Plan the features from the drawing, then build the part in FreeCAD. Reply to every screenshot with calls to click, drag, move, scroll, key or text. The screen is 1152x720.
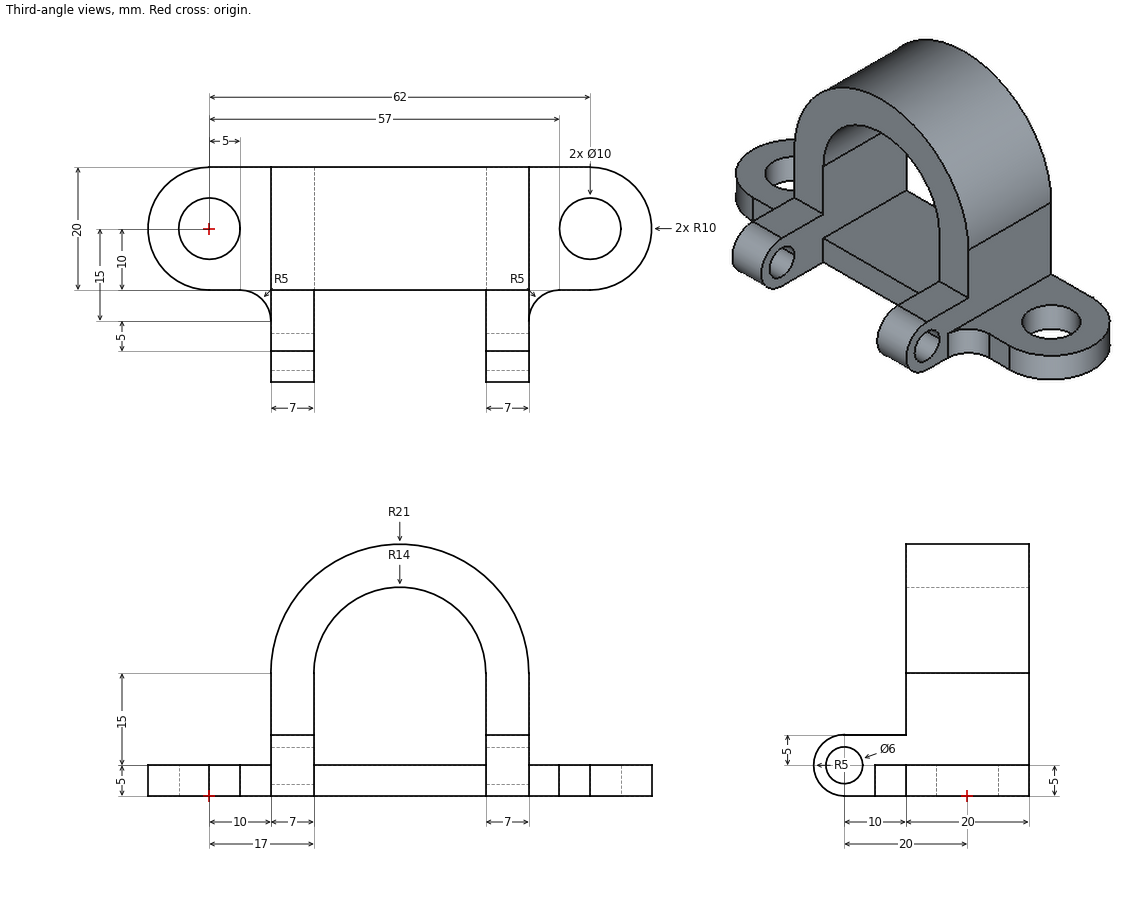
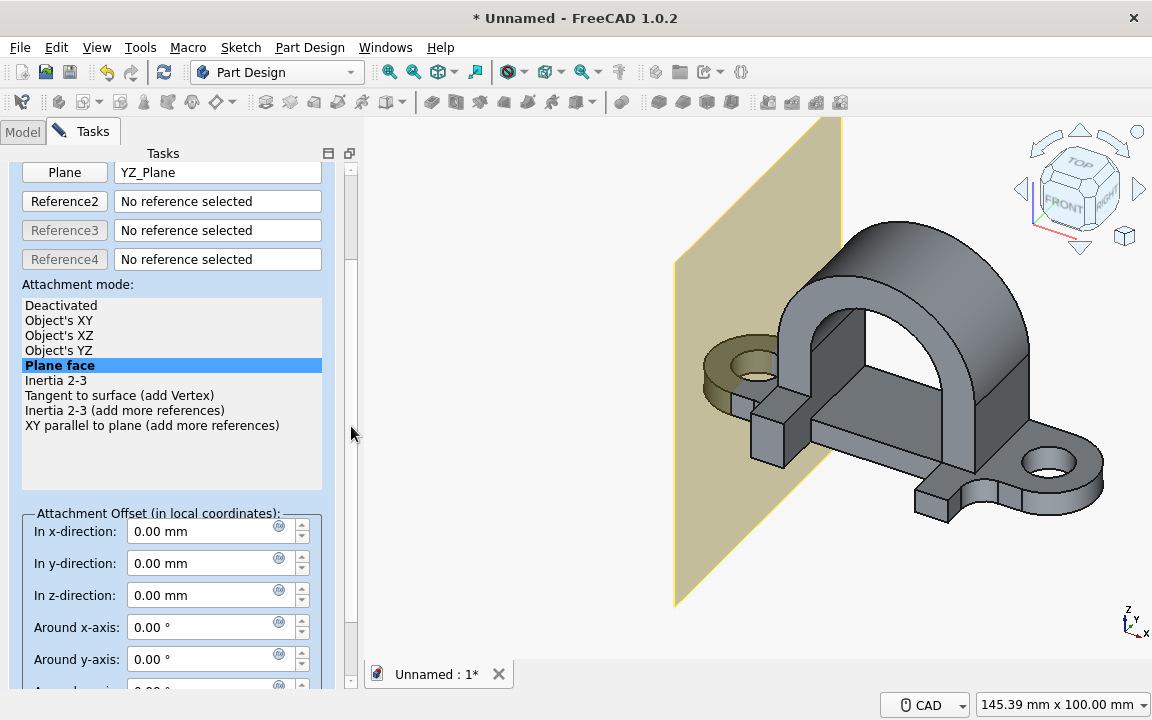
triple_click(210, 595)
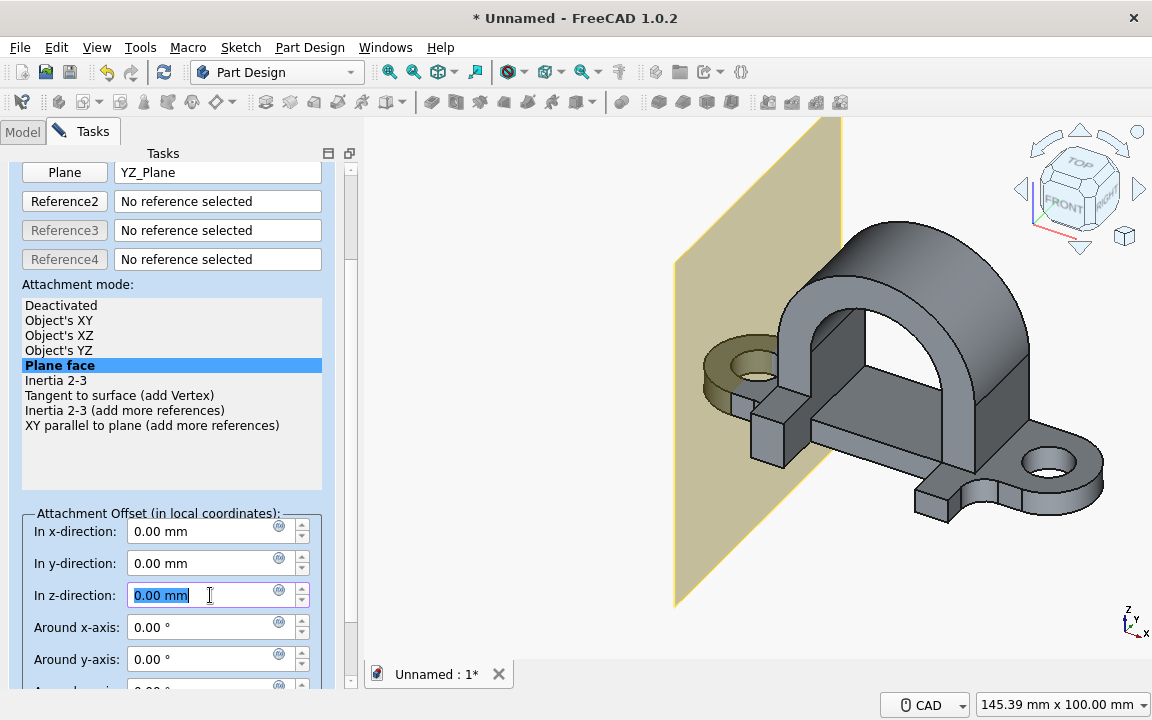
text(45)
key(Tab)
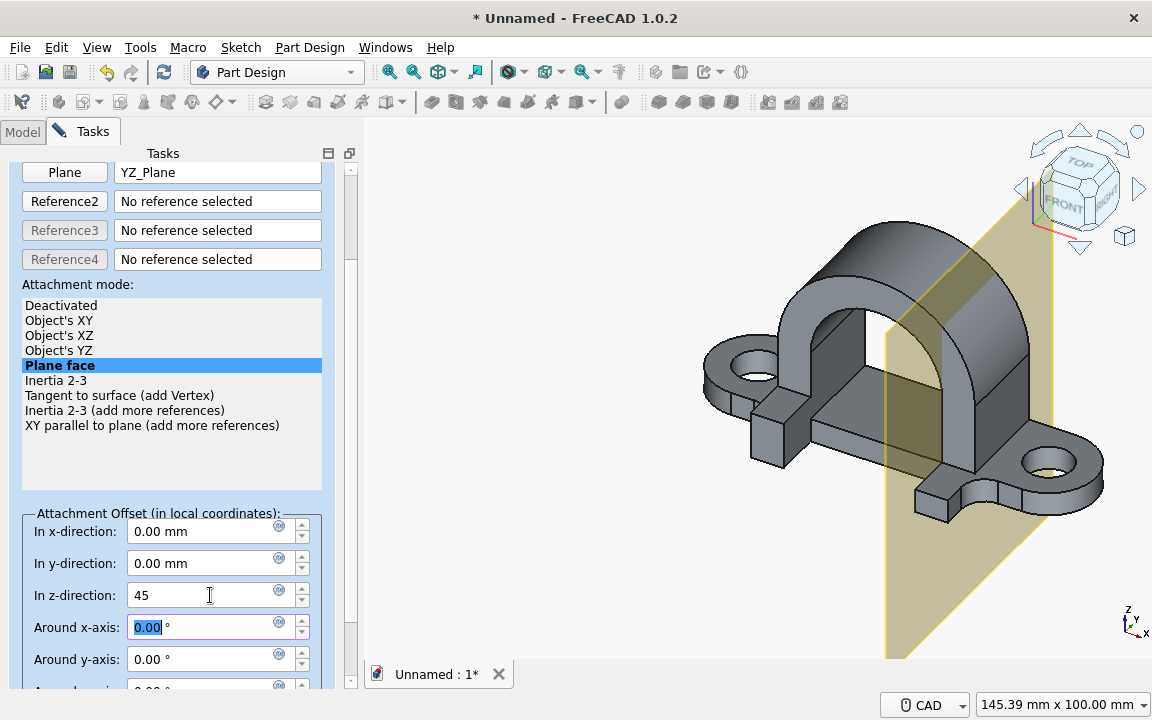
scroll(351, 426, up, 3)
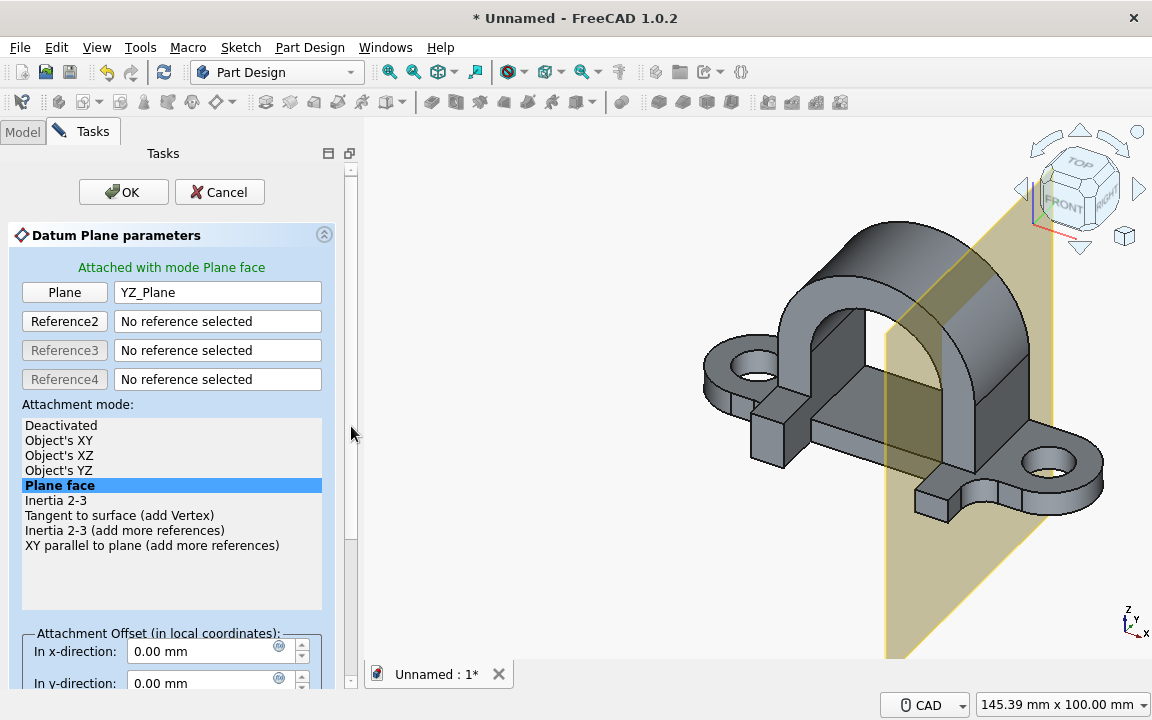
click(124, 192)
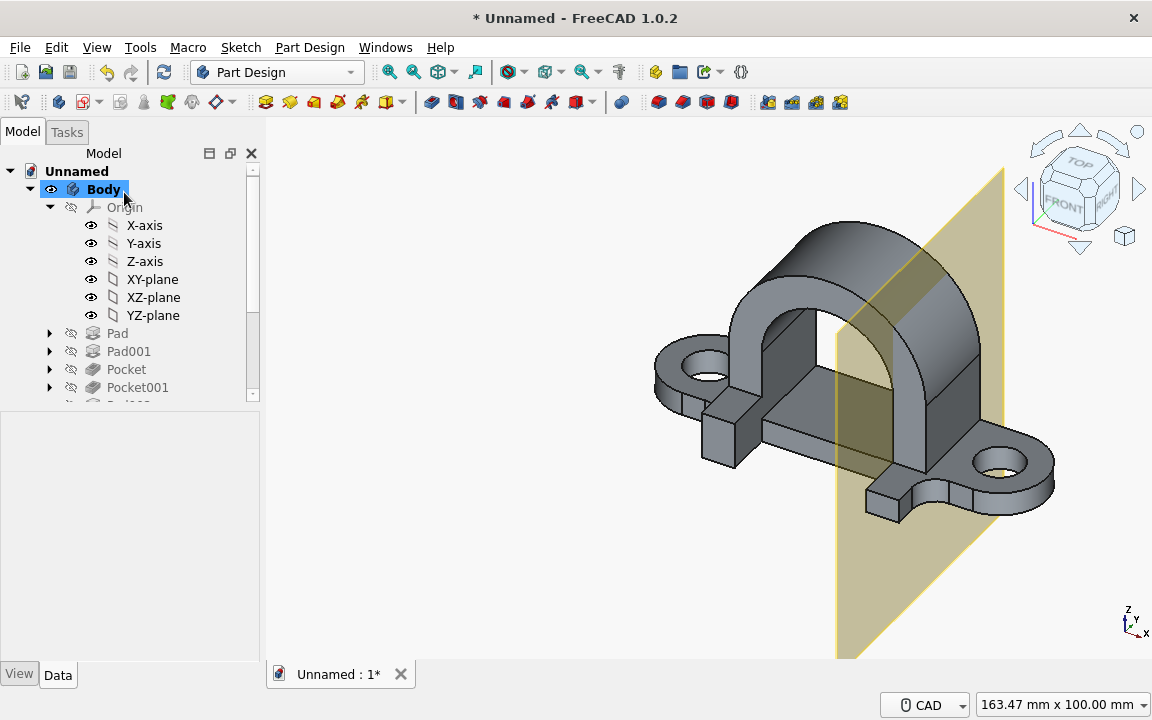
scroll(100, 275, down, 3)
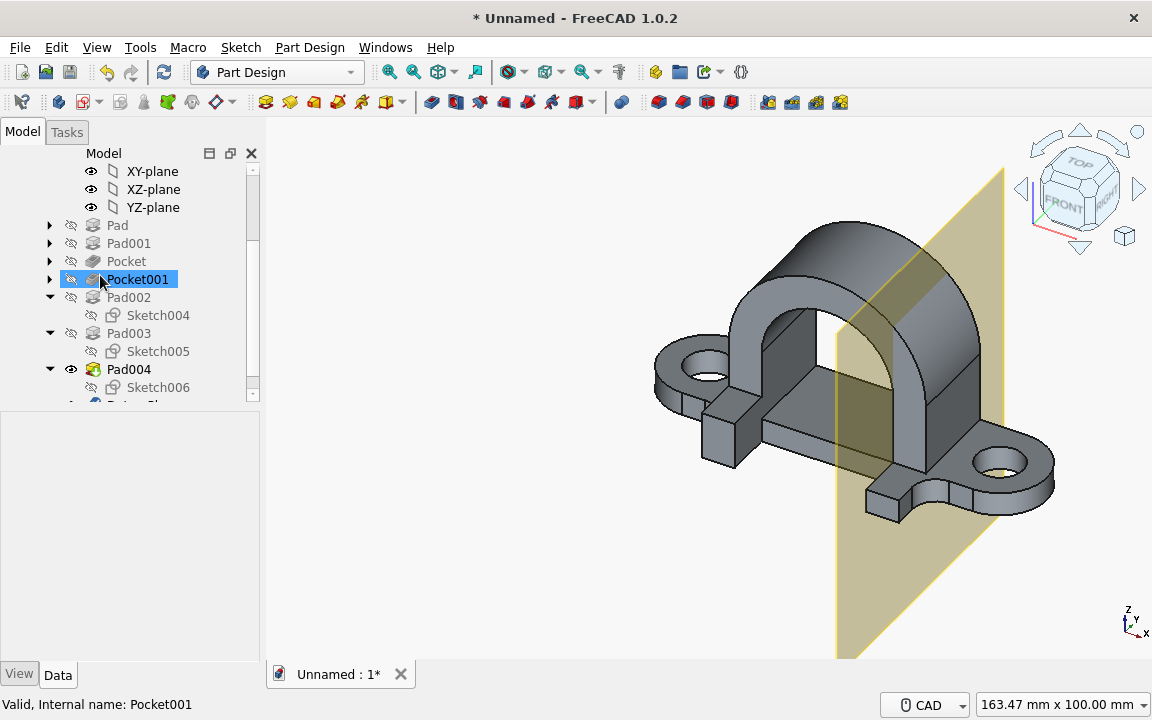
click(116, 387)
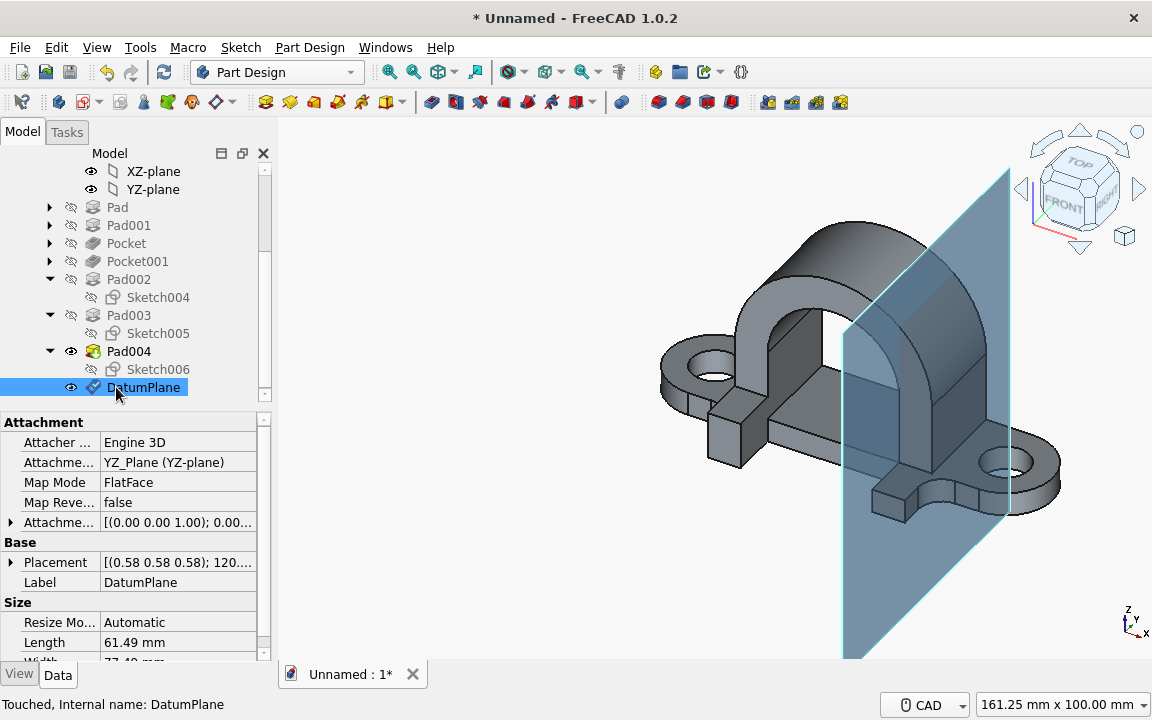
click(84, 102)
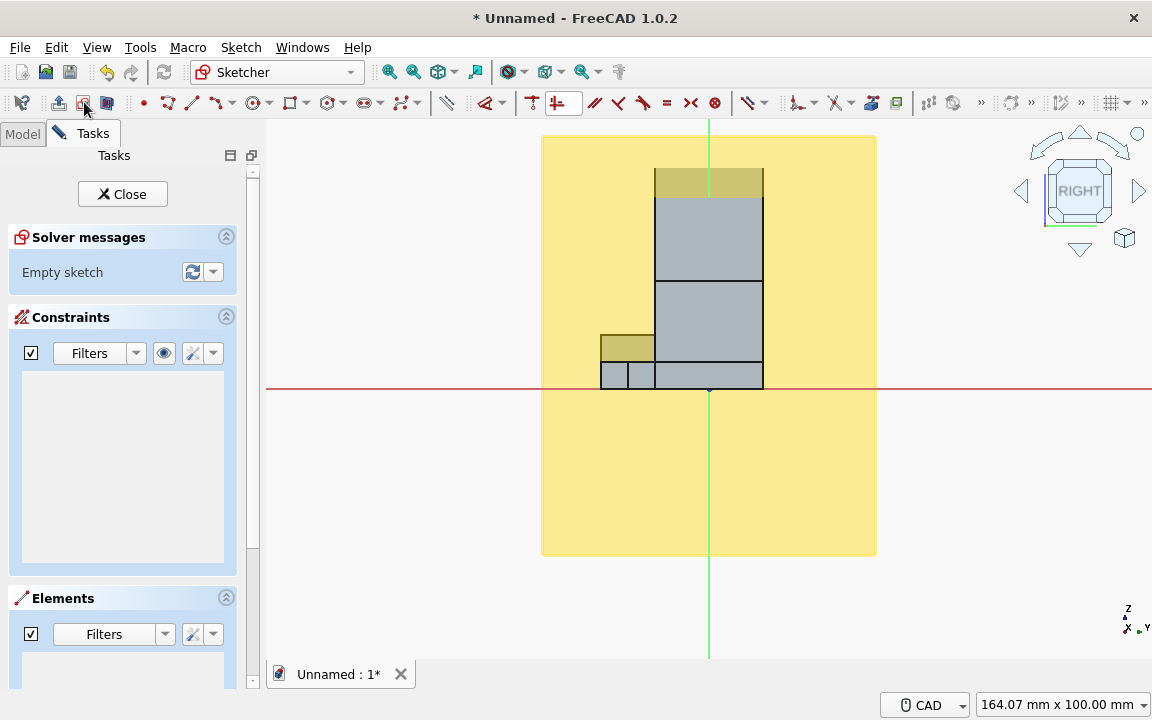
click(108, 104)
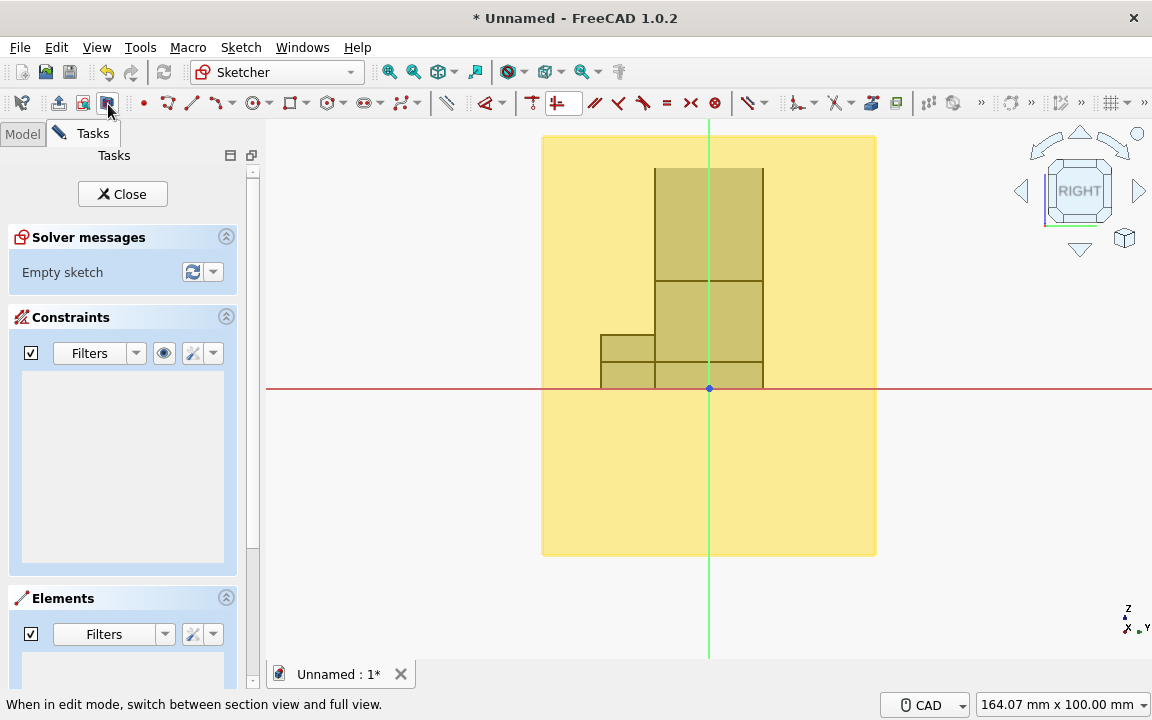
scroll(659, 355, up, 8)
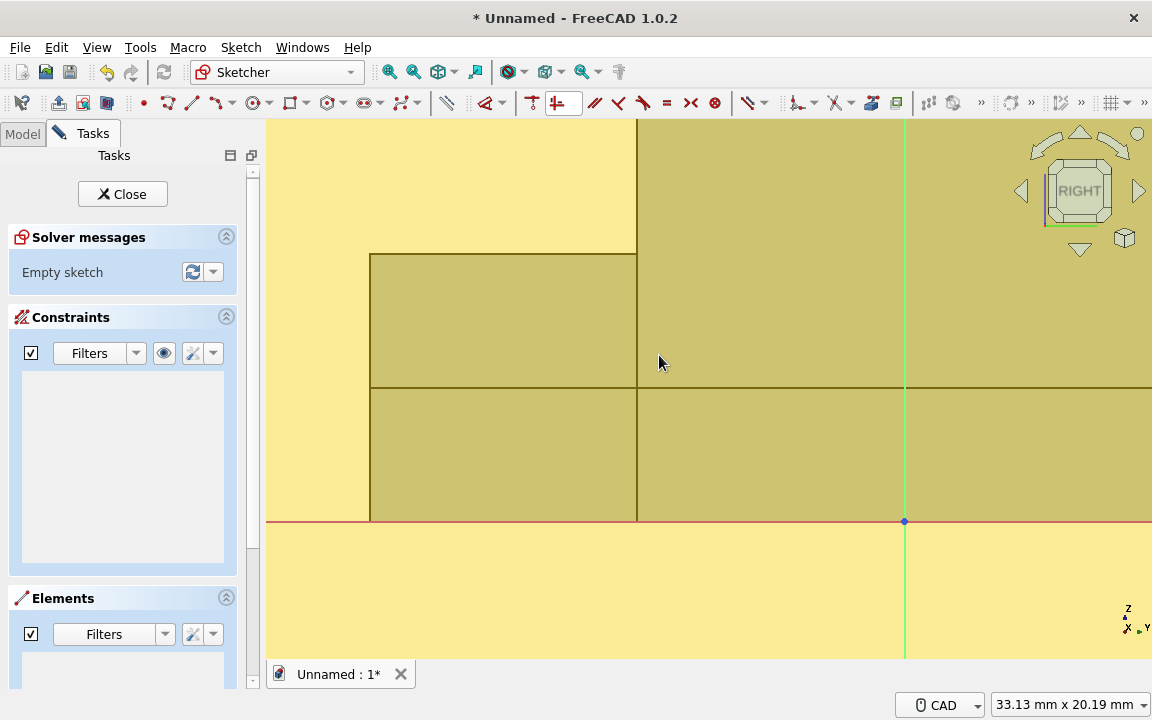
key(g)
key(r)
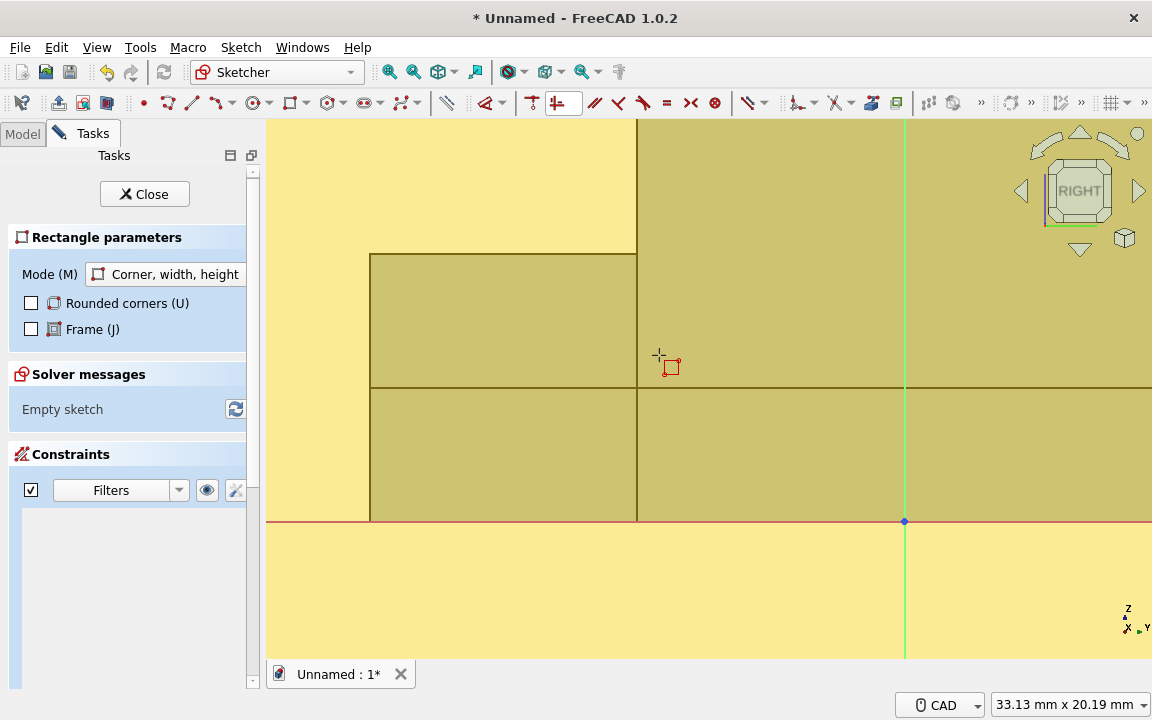
click(370, 254)
move(637, 388)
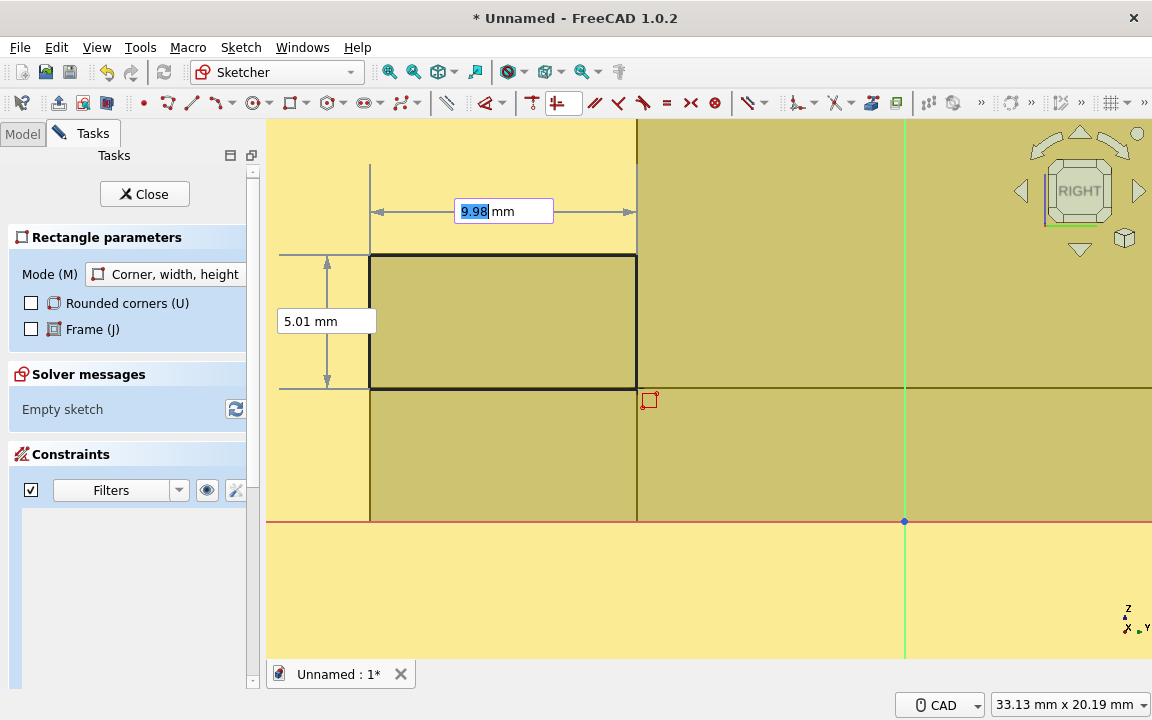
text(10)
key(Tab)
text(5)
key(Return)
key(Escape)